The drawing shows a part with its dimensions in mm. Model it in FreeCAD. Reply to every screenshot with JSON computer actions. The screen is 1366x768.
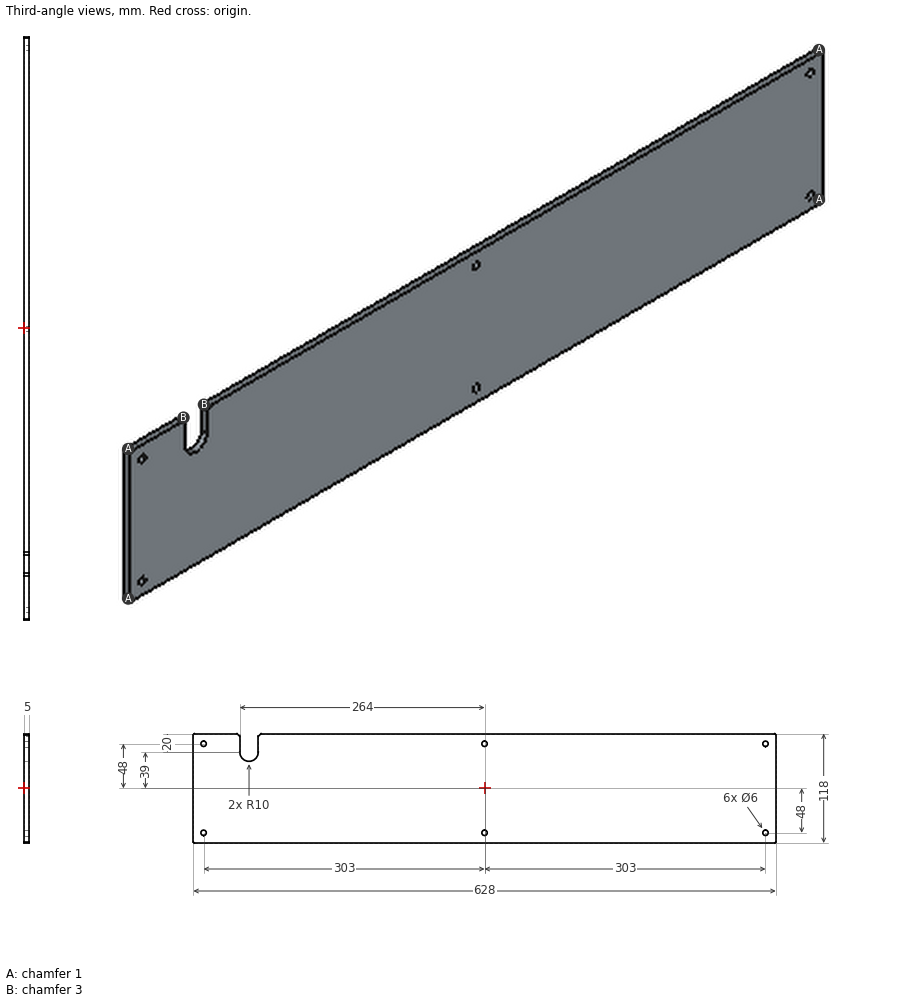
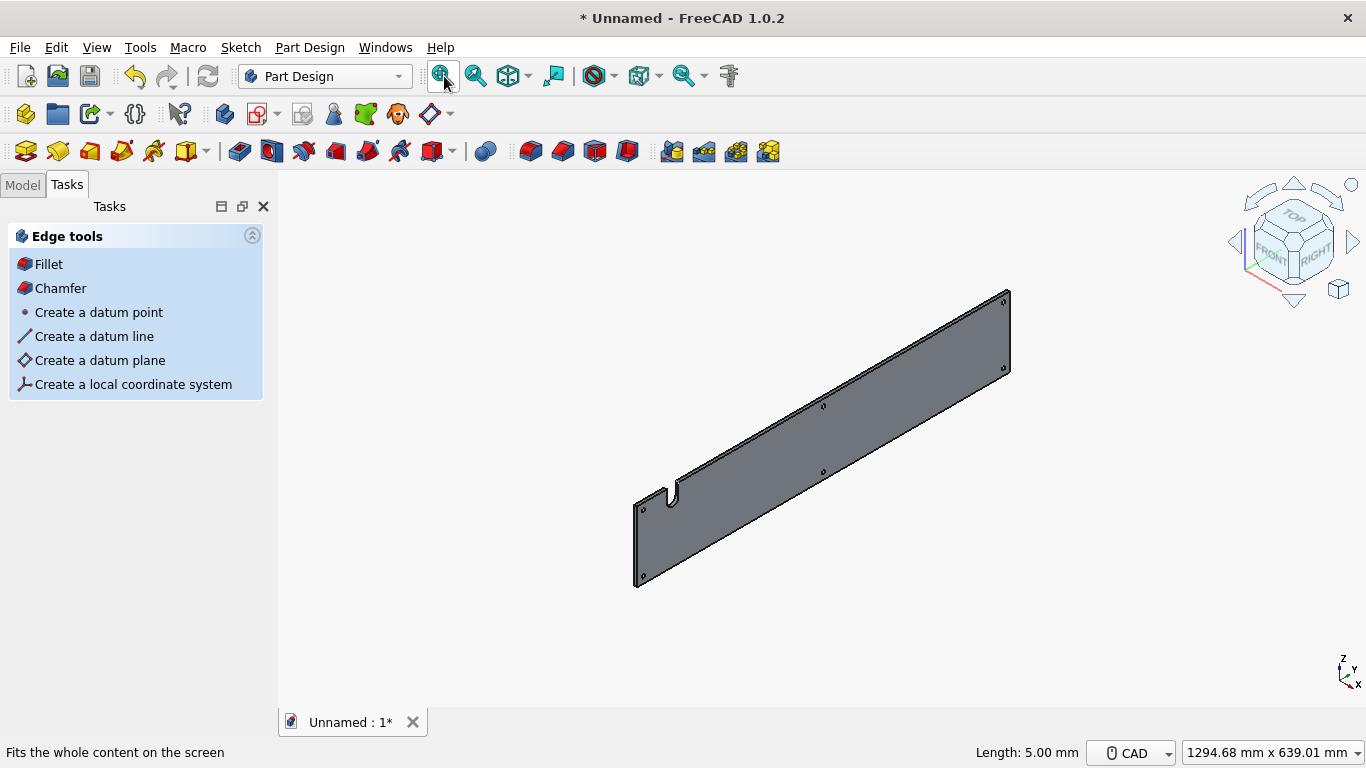
{"action": "key", "text": "2"}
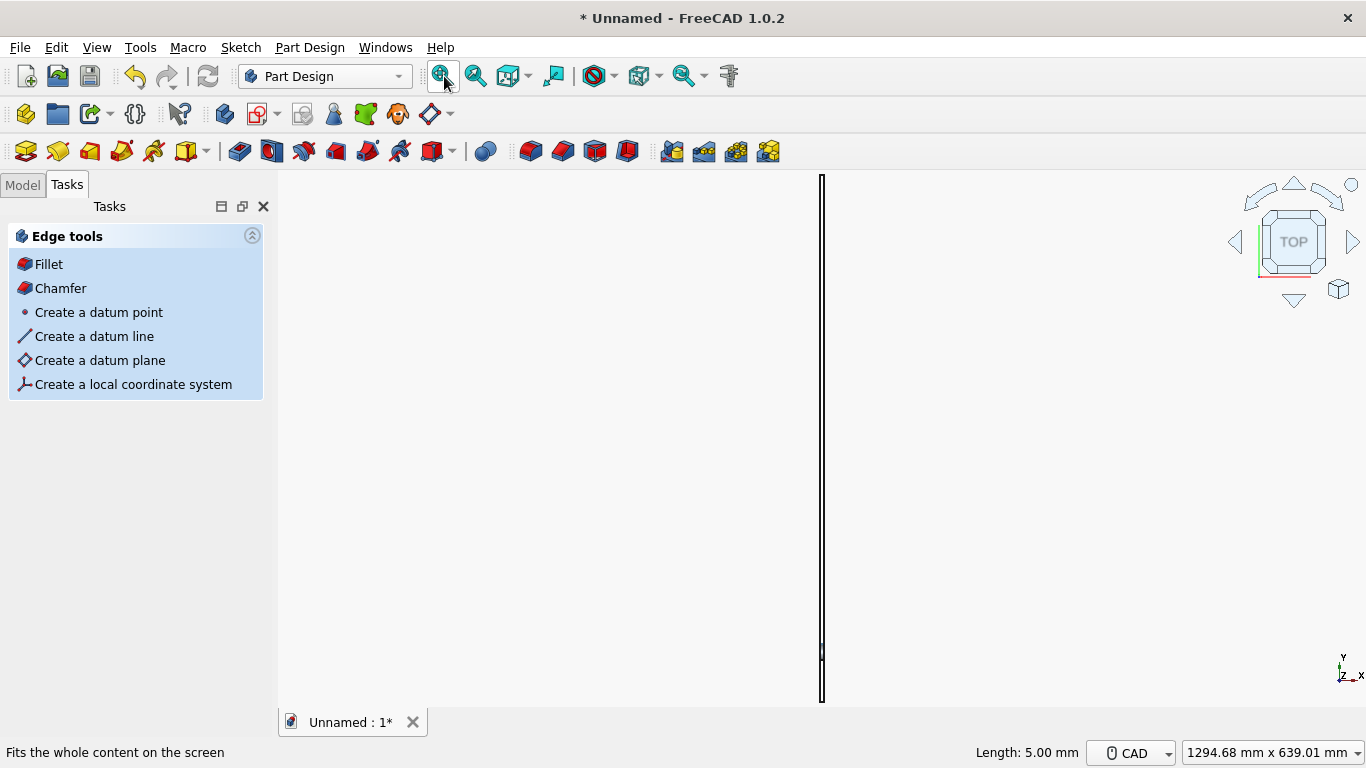
{"action": "scroll", "coordinate": [822, 659], "scroll_direction": "up", "scroll_amount": 12}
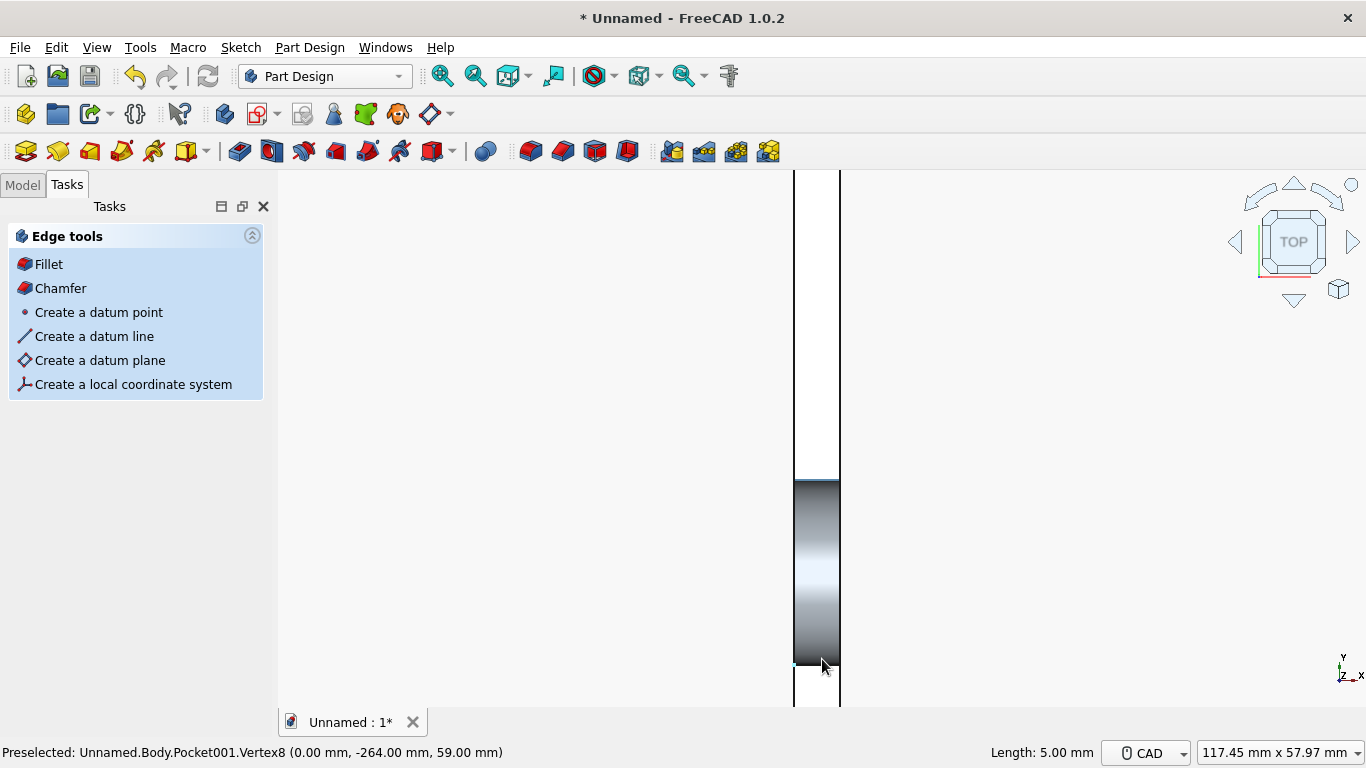
{"action": "left_click", "coordinate": [817, 664], "text": "ctrl"}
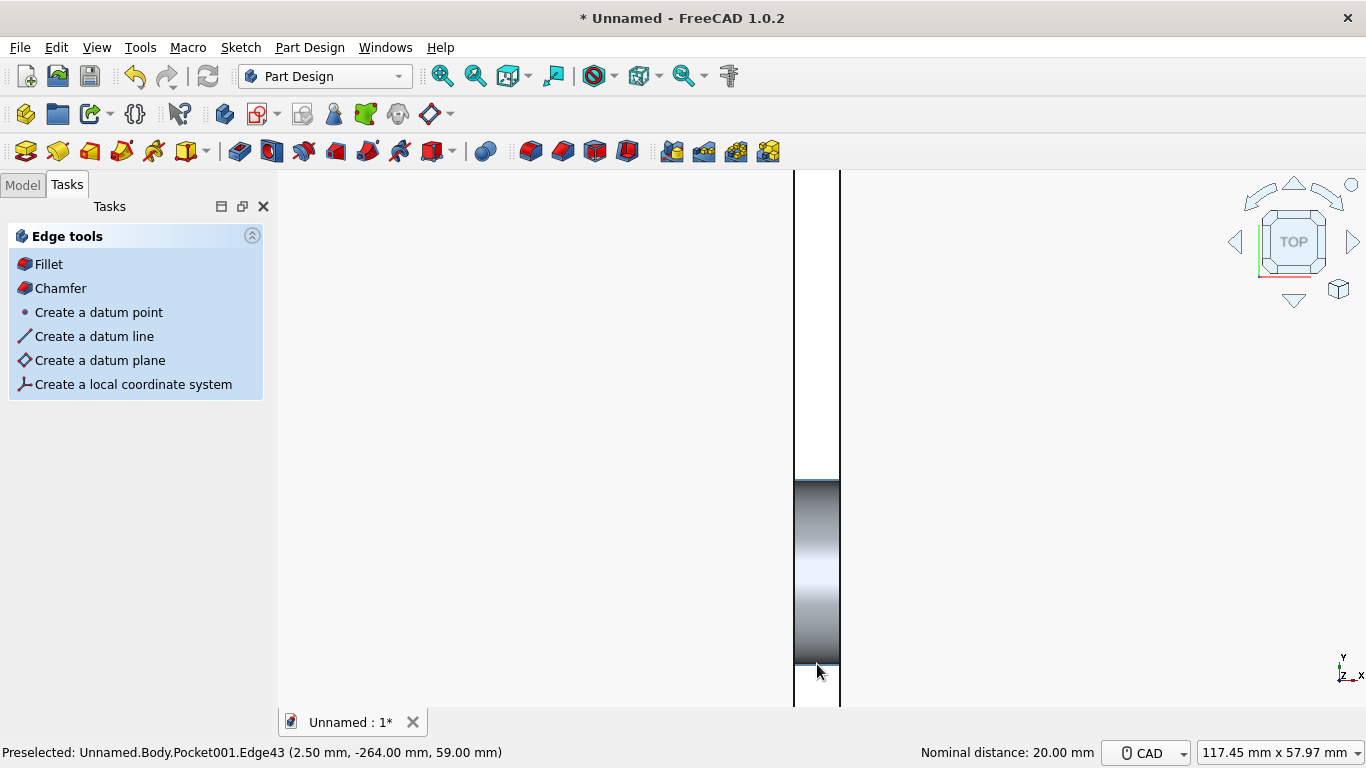
{"action": "left_click", "coordinate": [564, 152]}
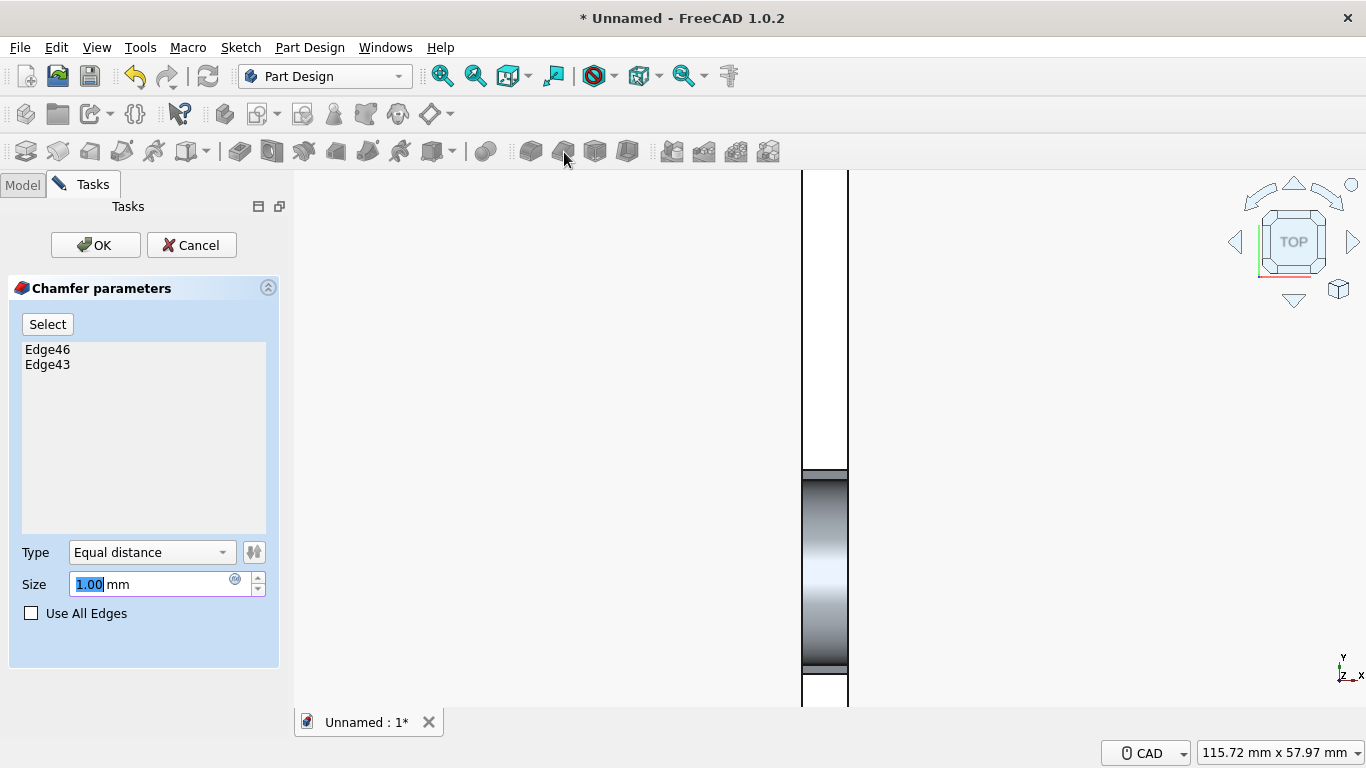
{"action": "type", "text": "3"}
{"action": "key", "text": "Tab"}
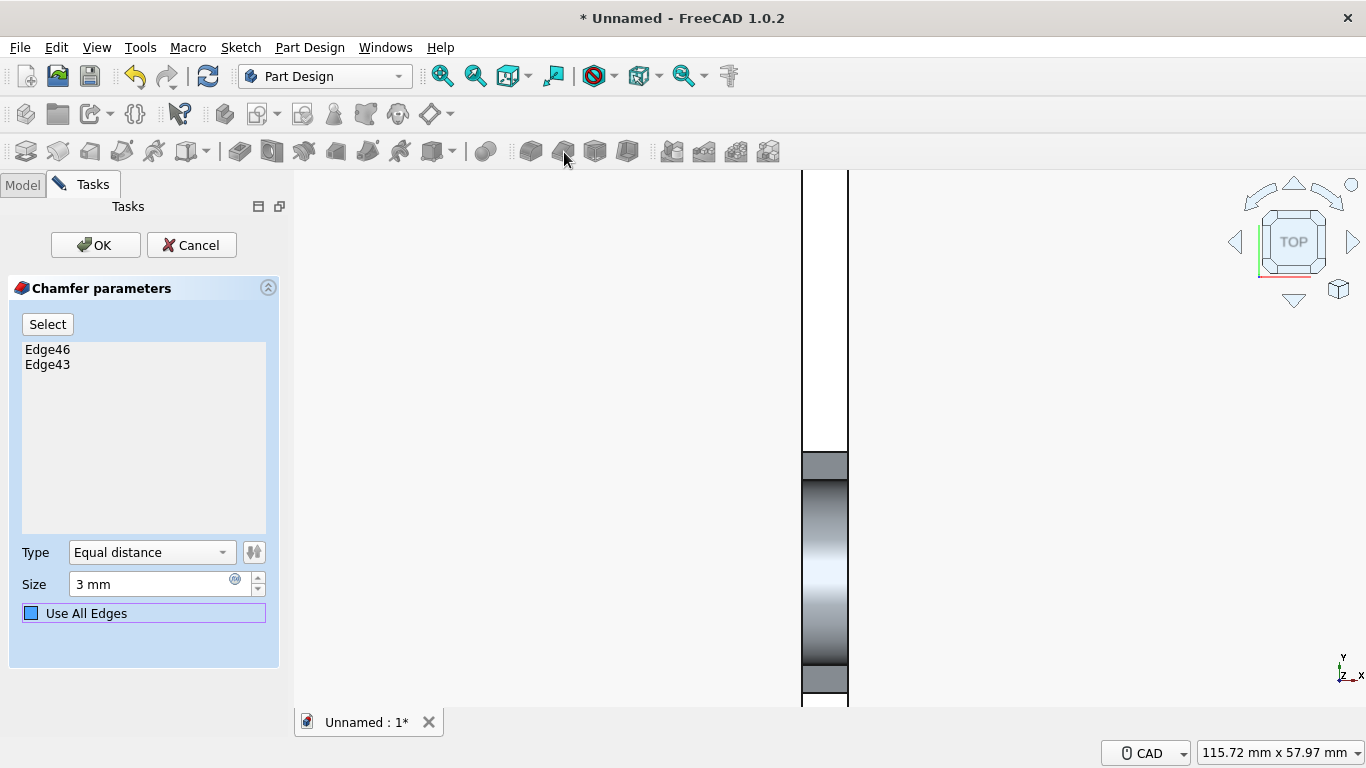
{"action": "left_click", "coordinate": [96, 245]}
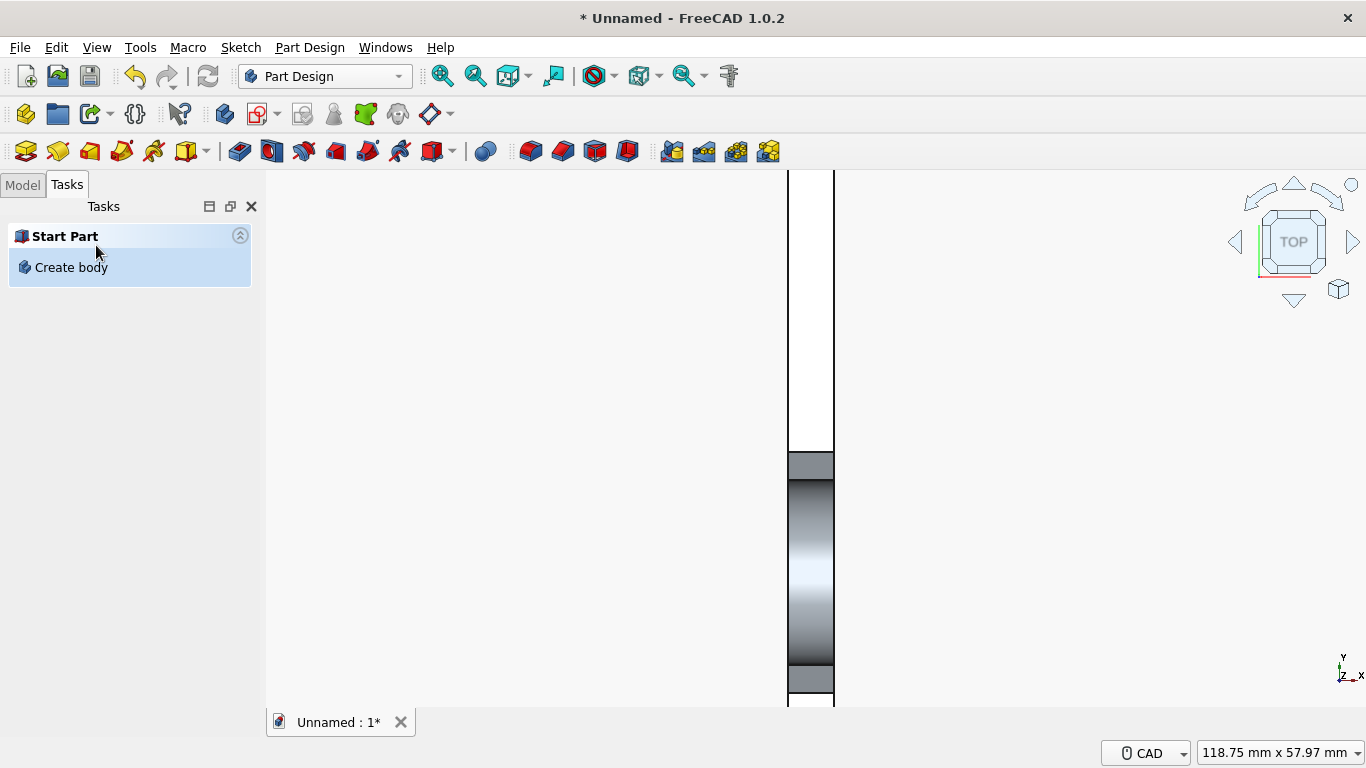
{"action": "key", "text": "0"}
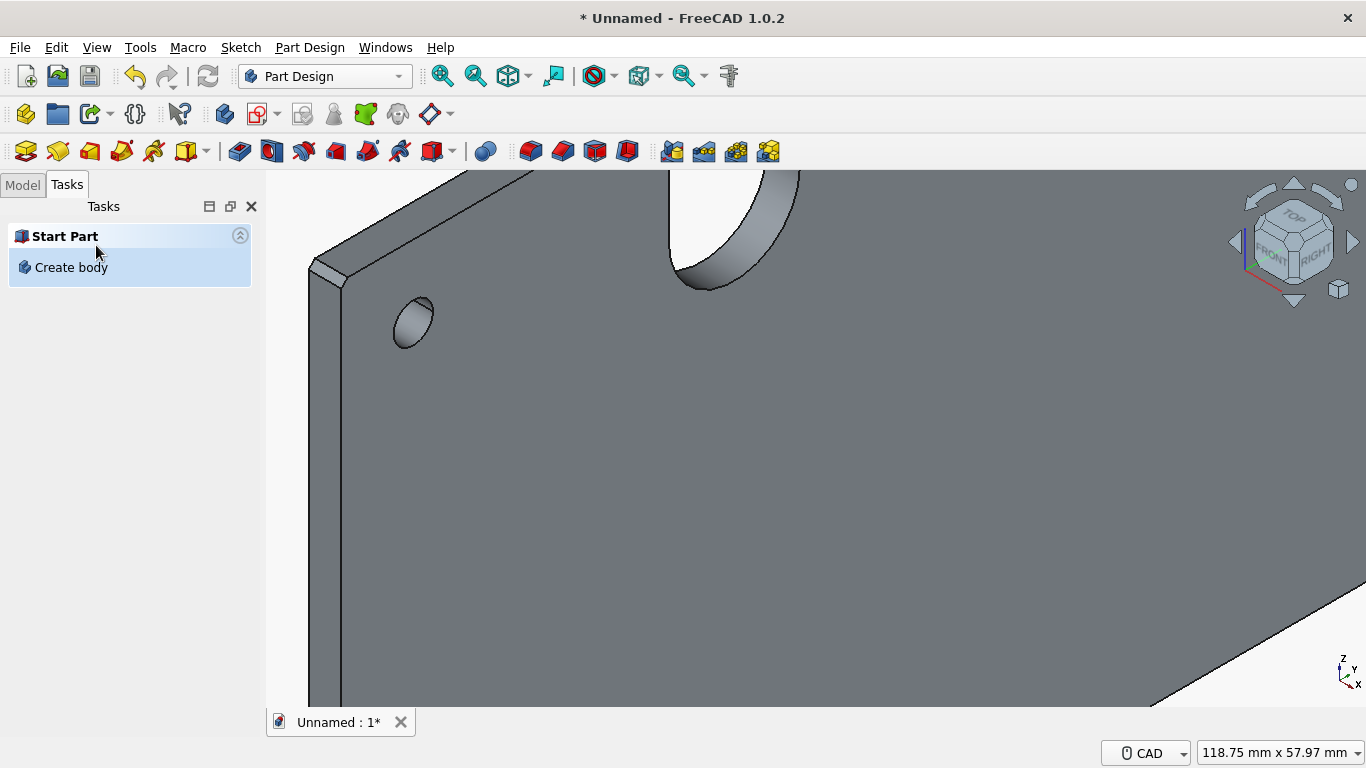
{"action": "key", "text": "v f"}